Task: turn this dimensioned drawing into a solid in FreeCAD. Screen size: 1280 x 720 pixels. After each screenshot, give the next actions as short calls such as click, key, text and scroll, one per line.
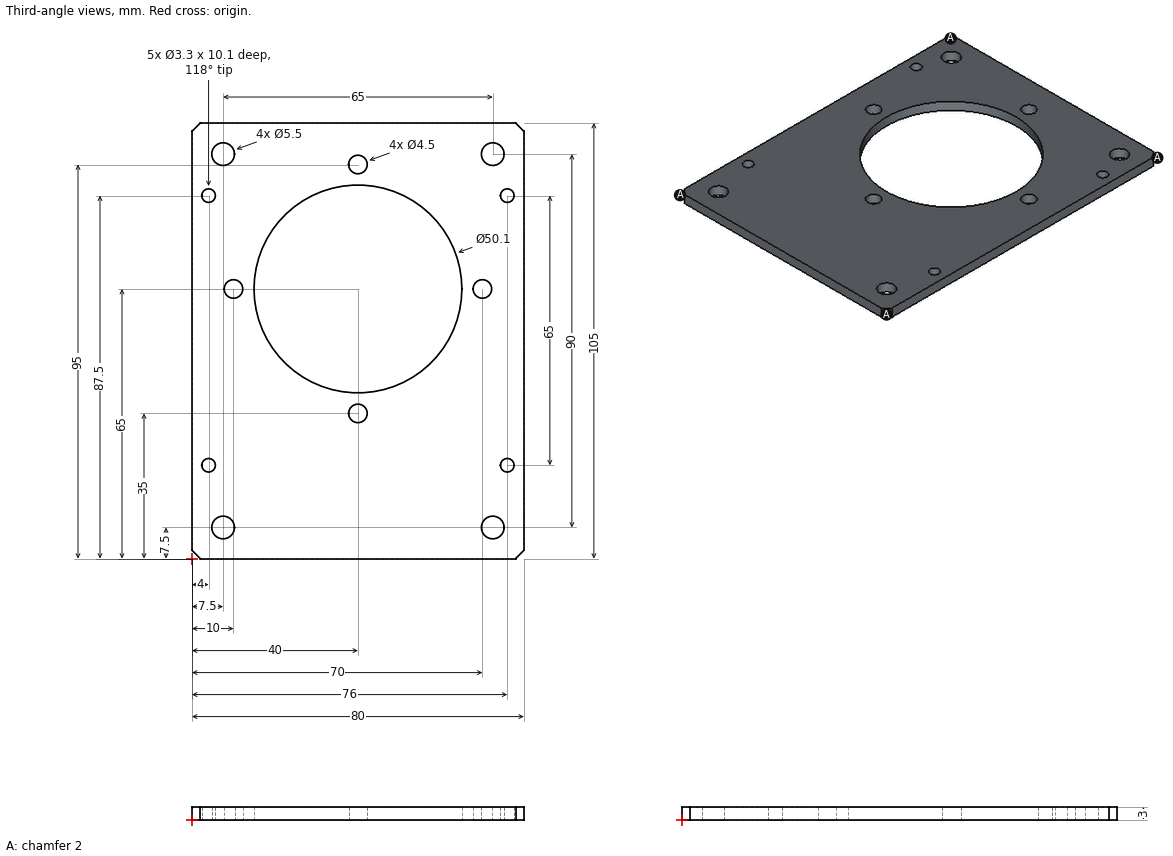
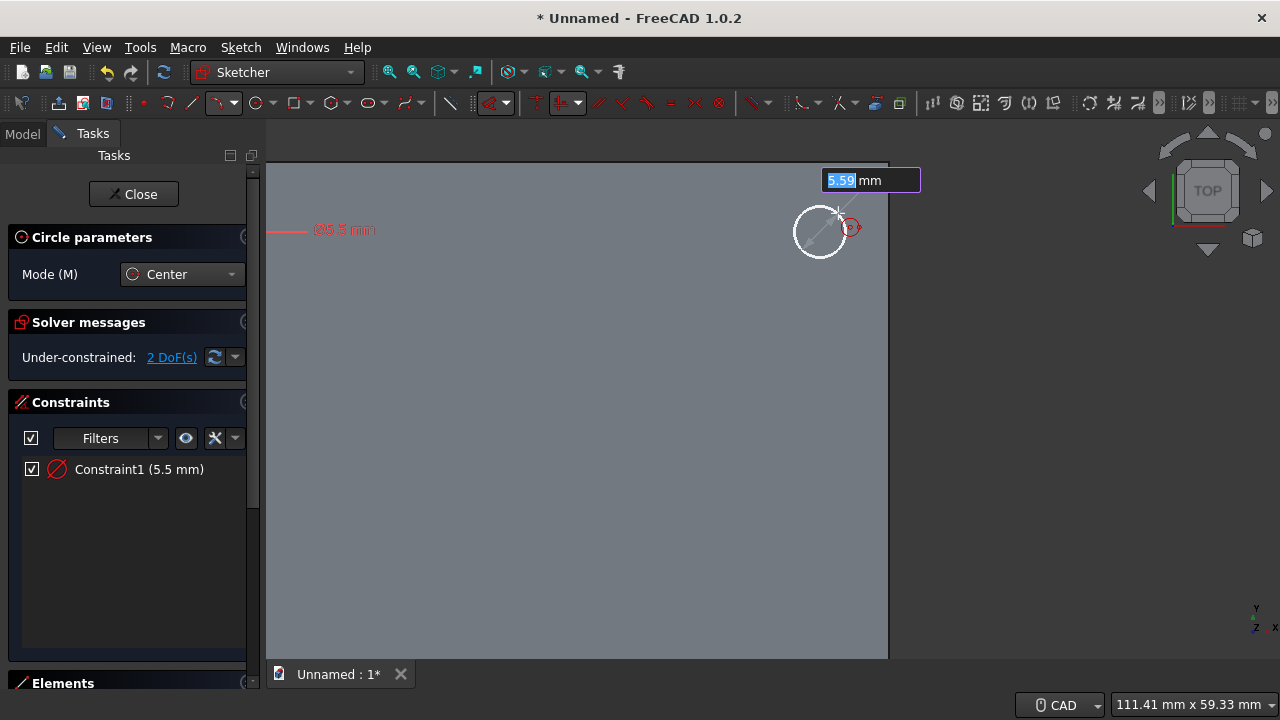
text(5.5)
key(Return)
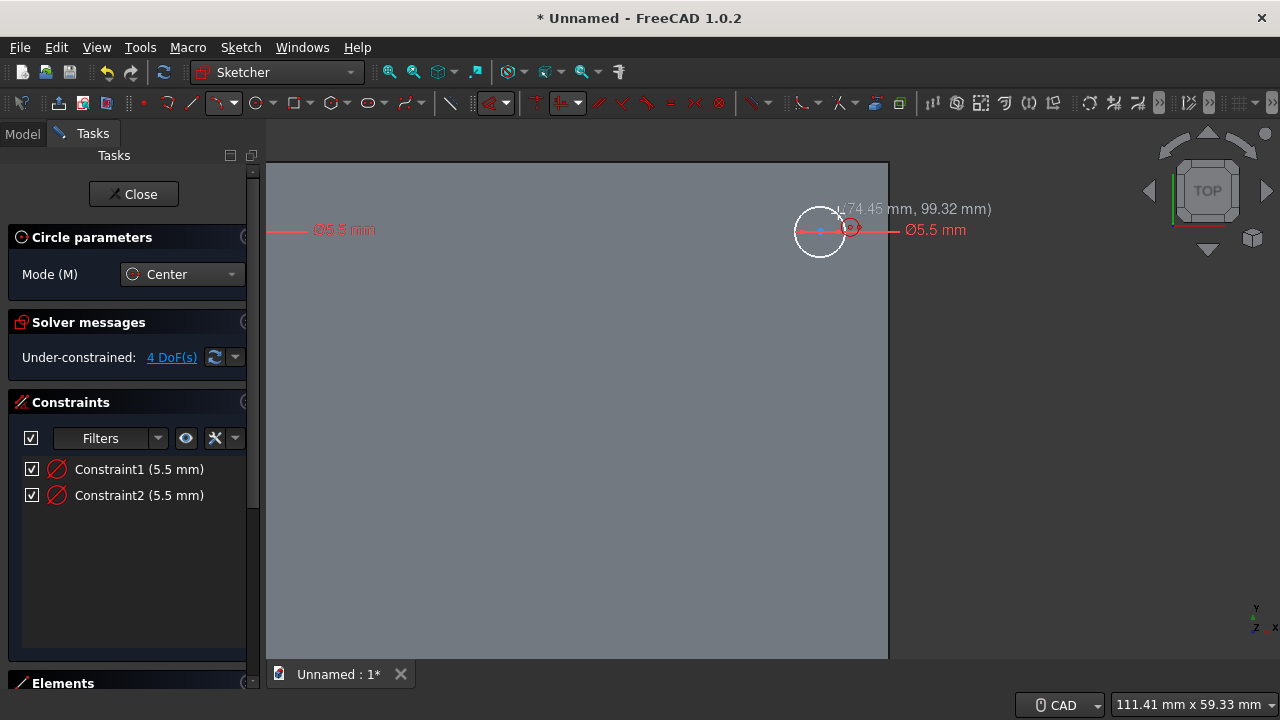
scroll(822, 230, down, 5)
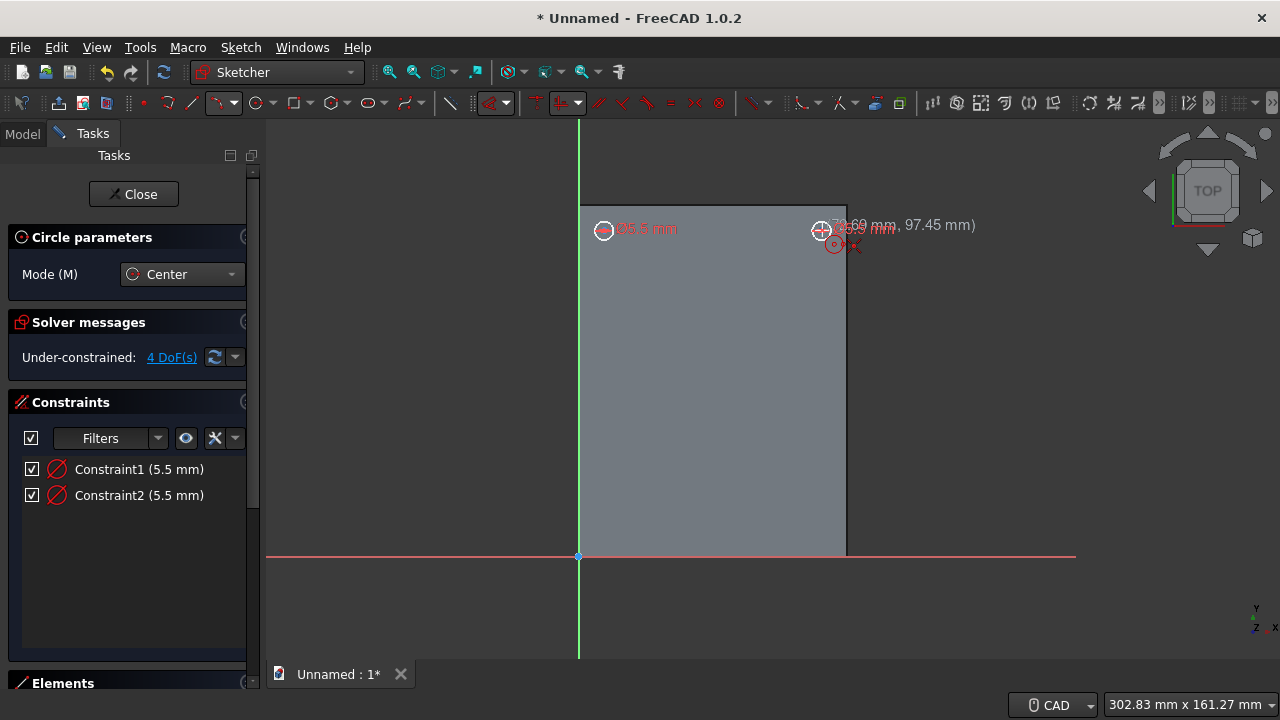
scroll(822, 532, up, 5)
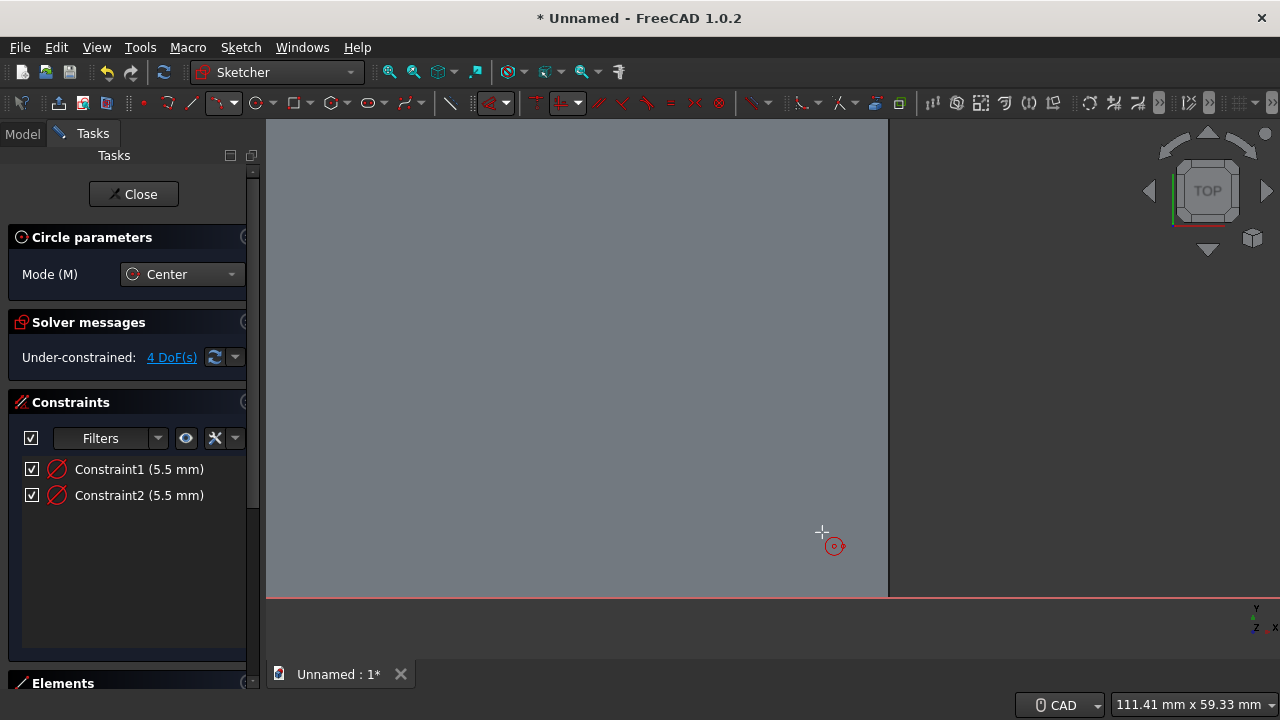
click(820, 530)
move(838, 512)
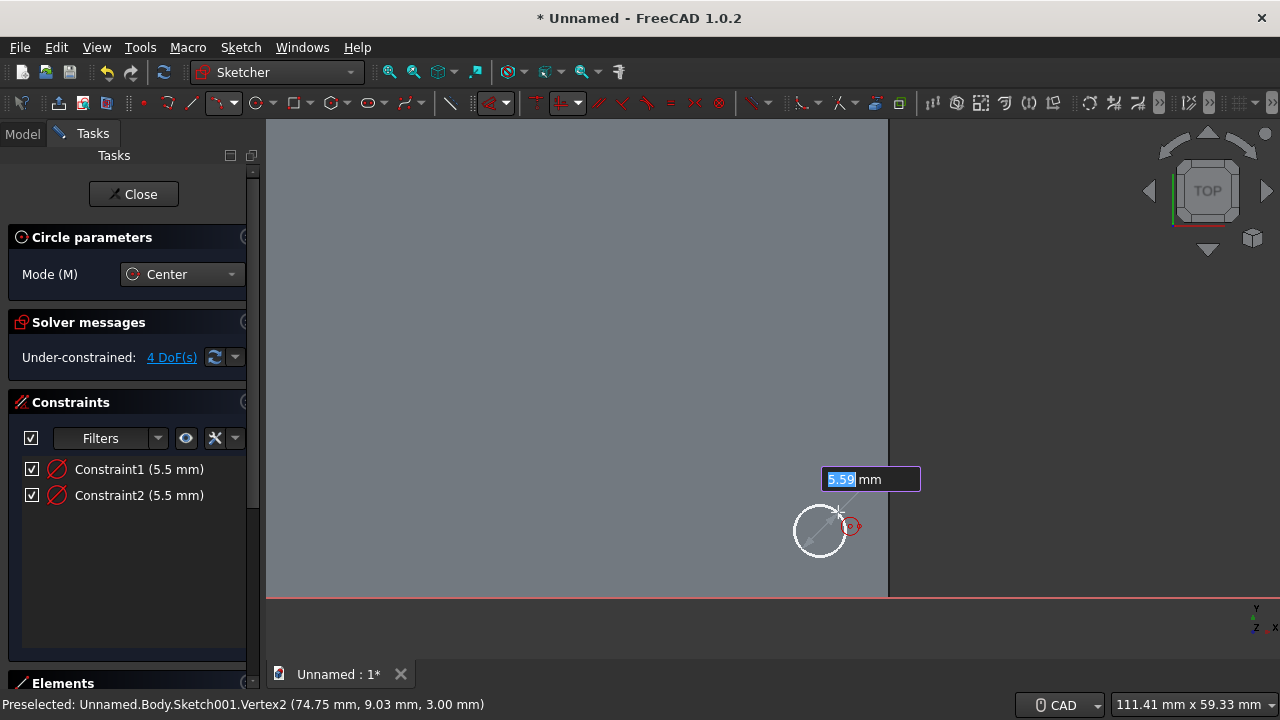
text(5.5)
key(Return)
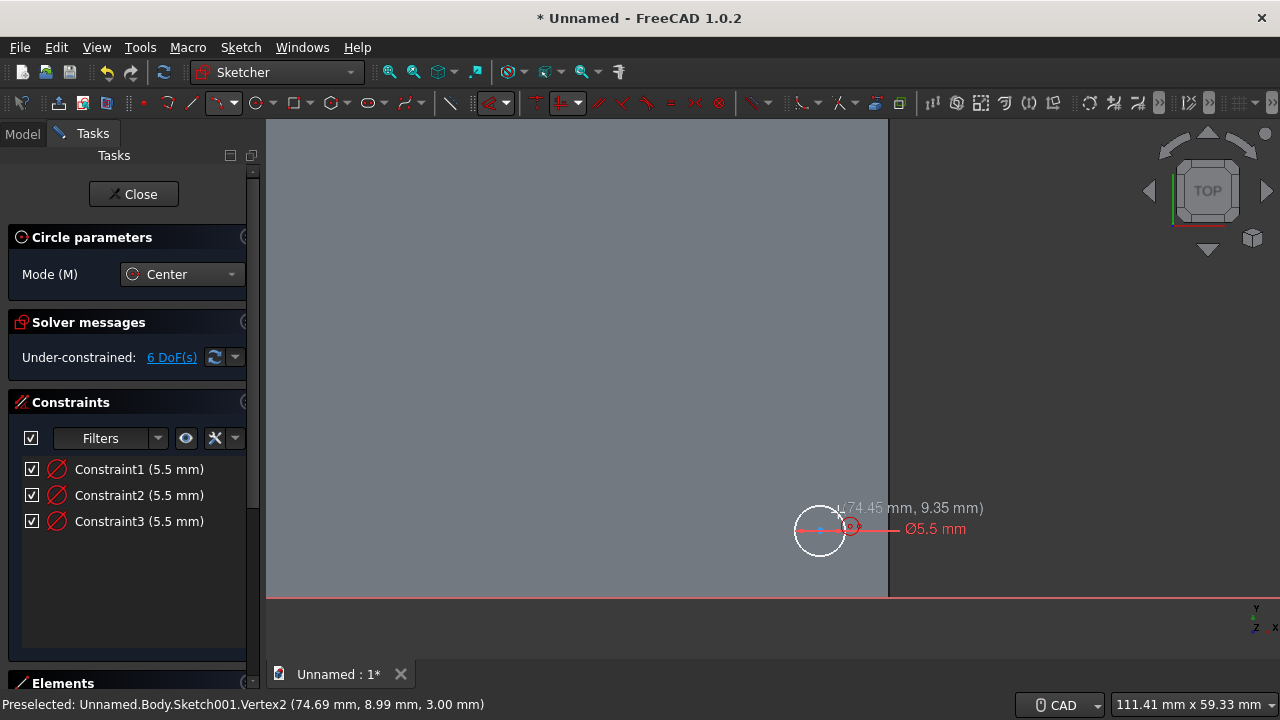
scroll(822, 533, down, 5)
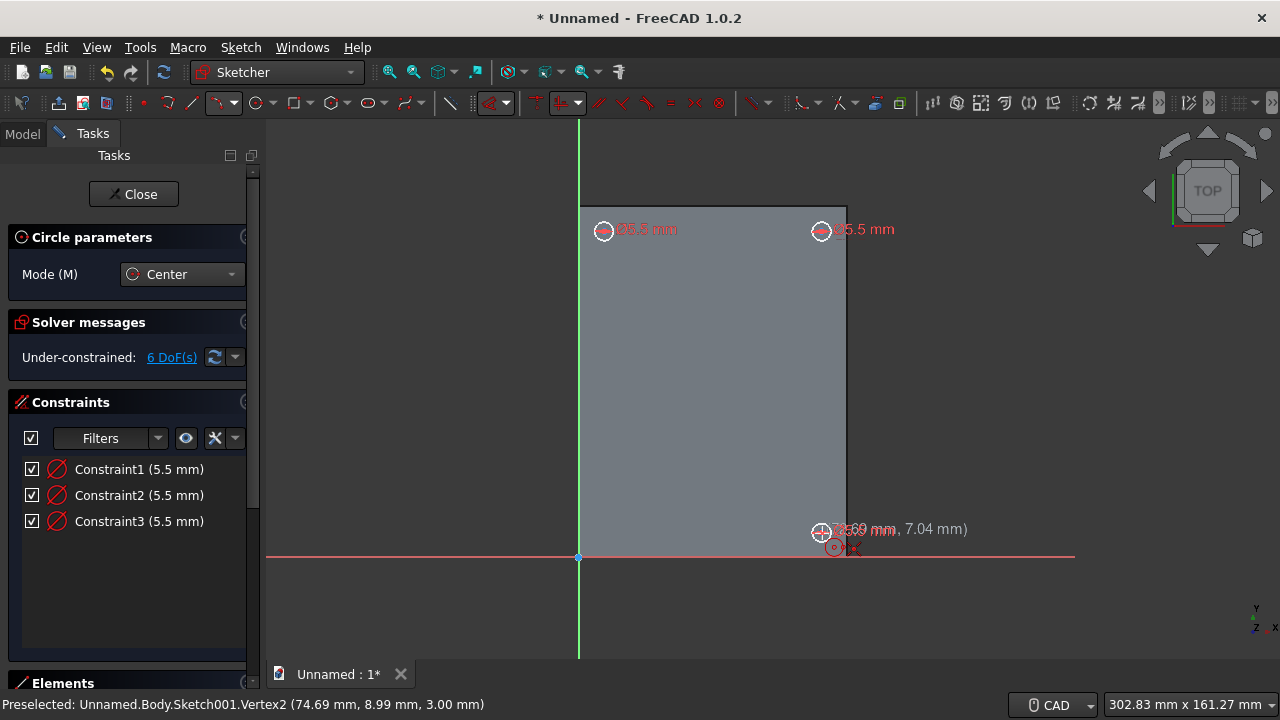
scroll(604, 532, up, 5)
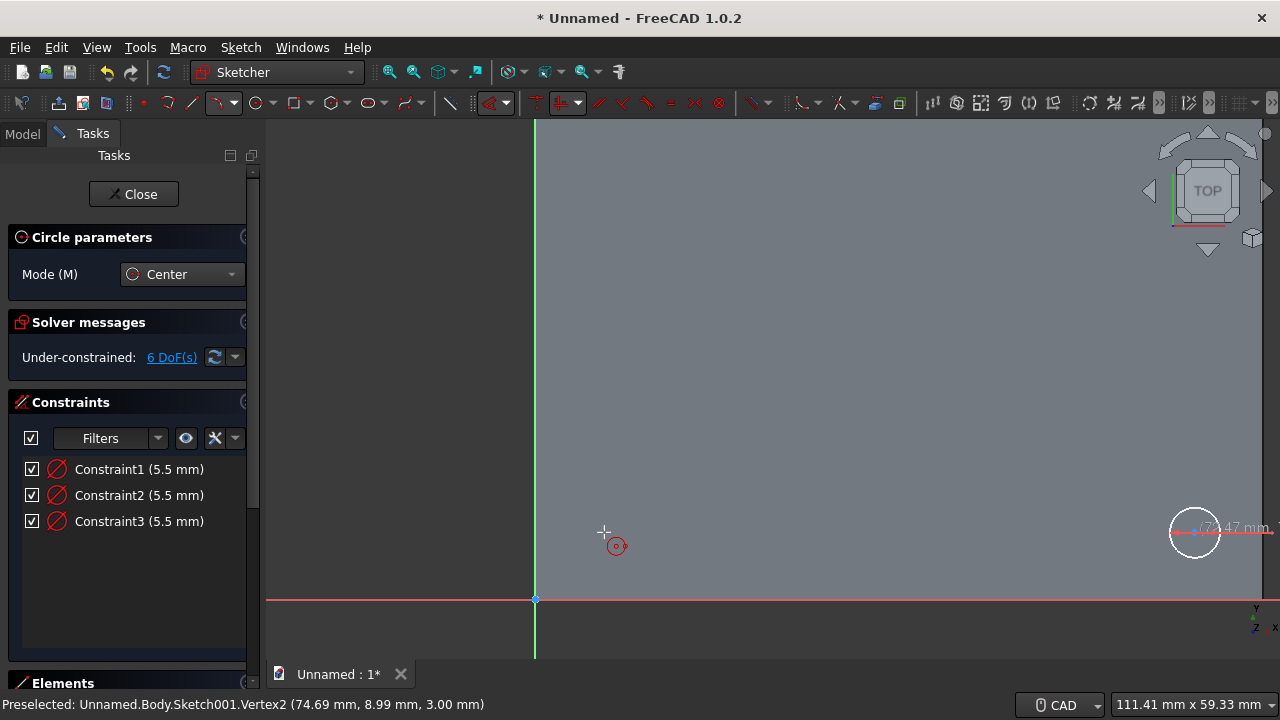
click(604, 532)
move(621, 514)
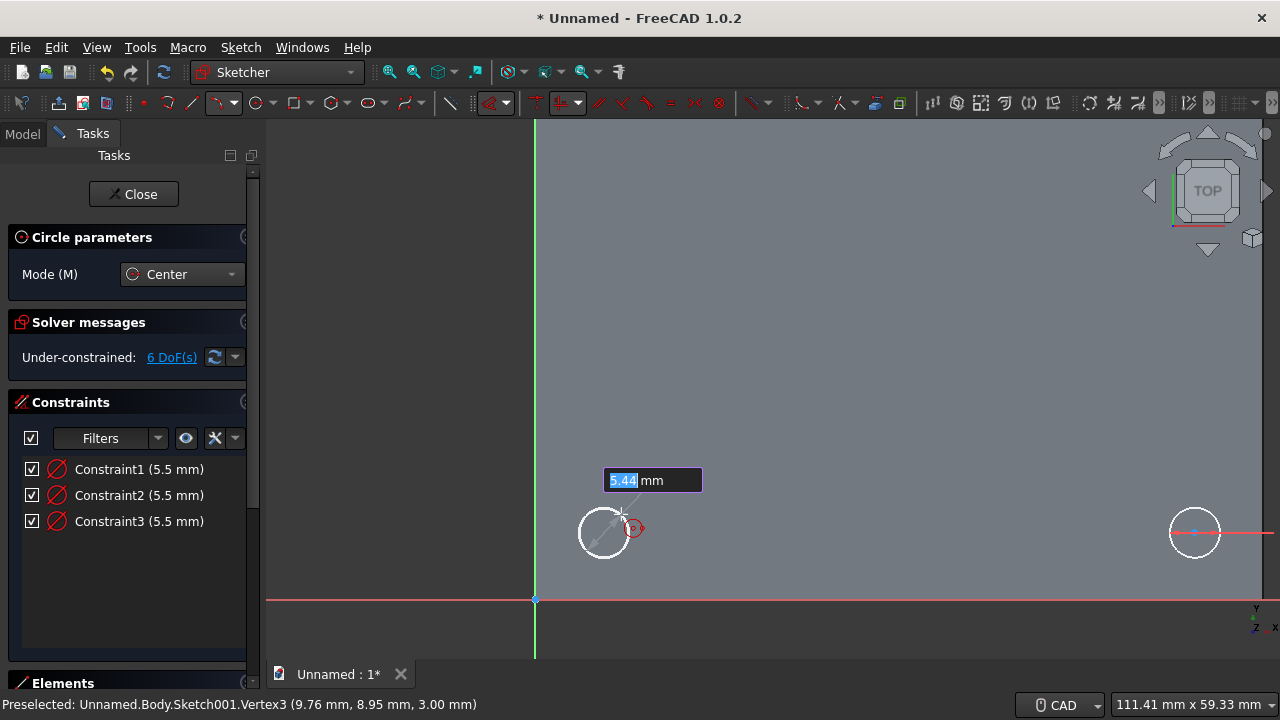
text(5.5)
key(Return)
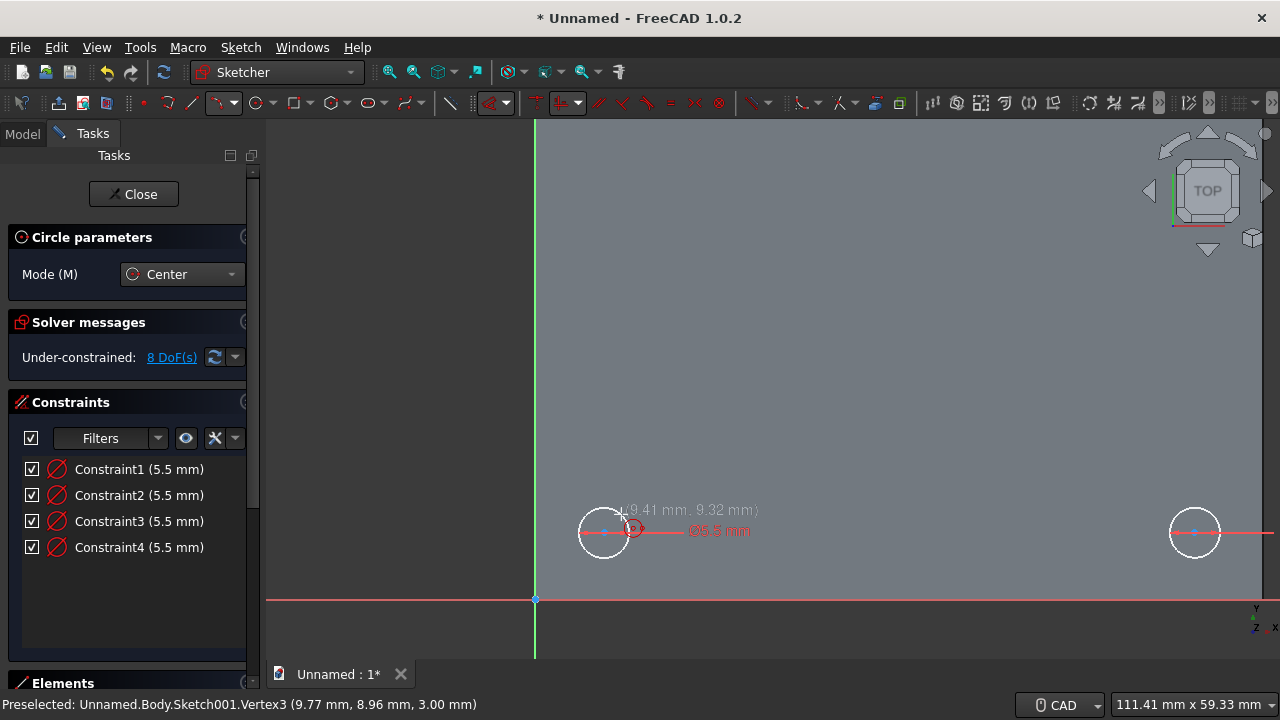
scroll(604, 532, down, 5)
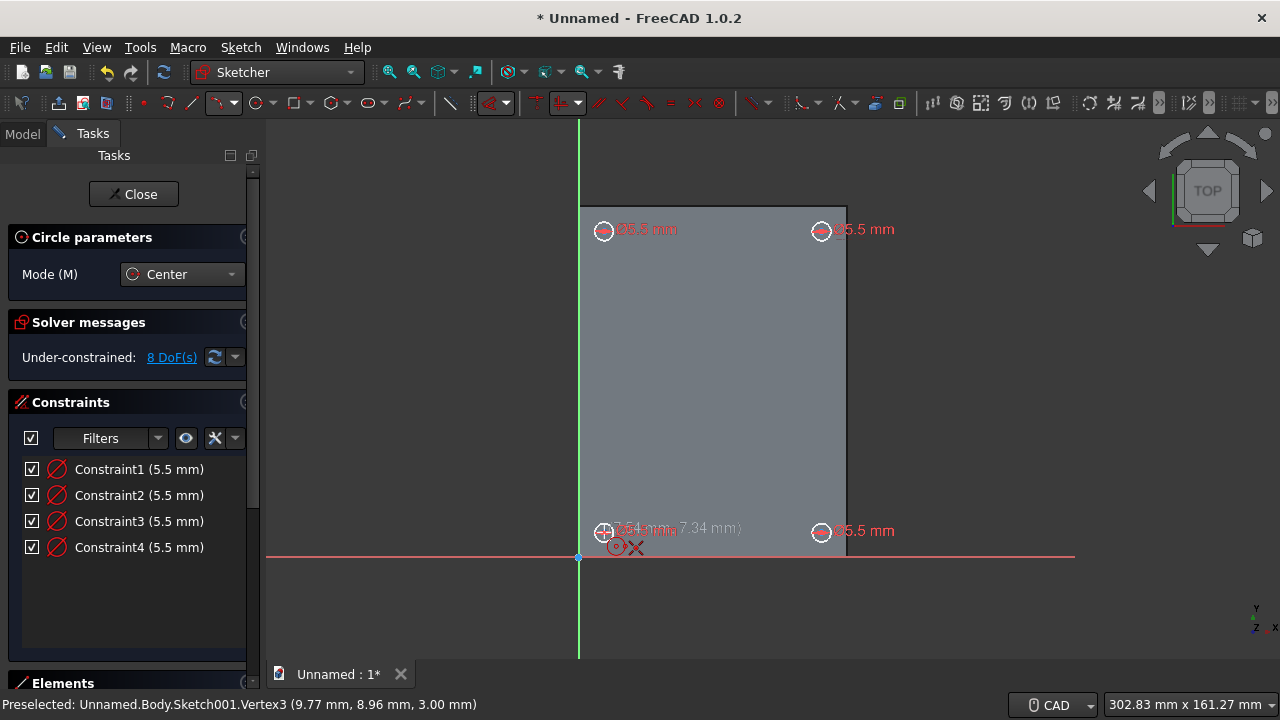
click(713, 340)
move(772, 280)